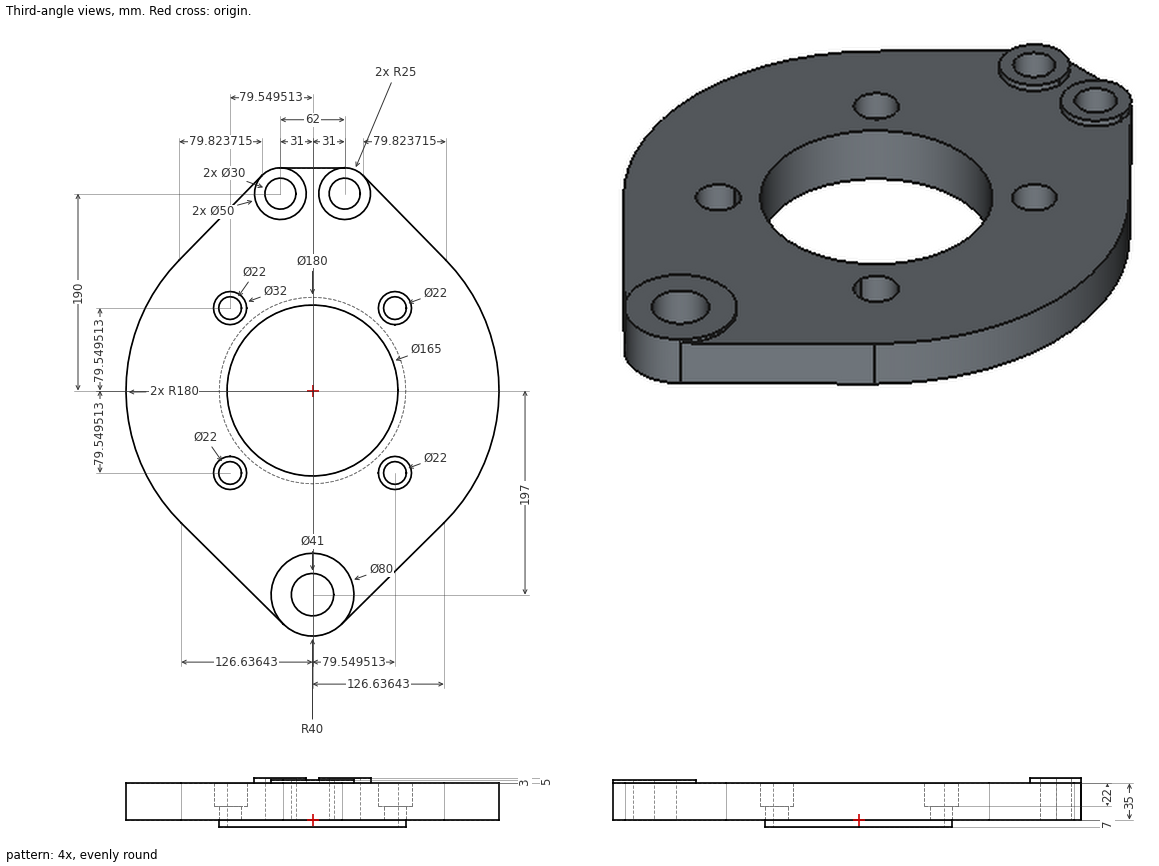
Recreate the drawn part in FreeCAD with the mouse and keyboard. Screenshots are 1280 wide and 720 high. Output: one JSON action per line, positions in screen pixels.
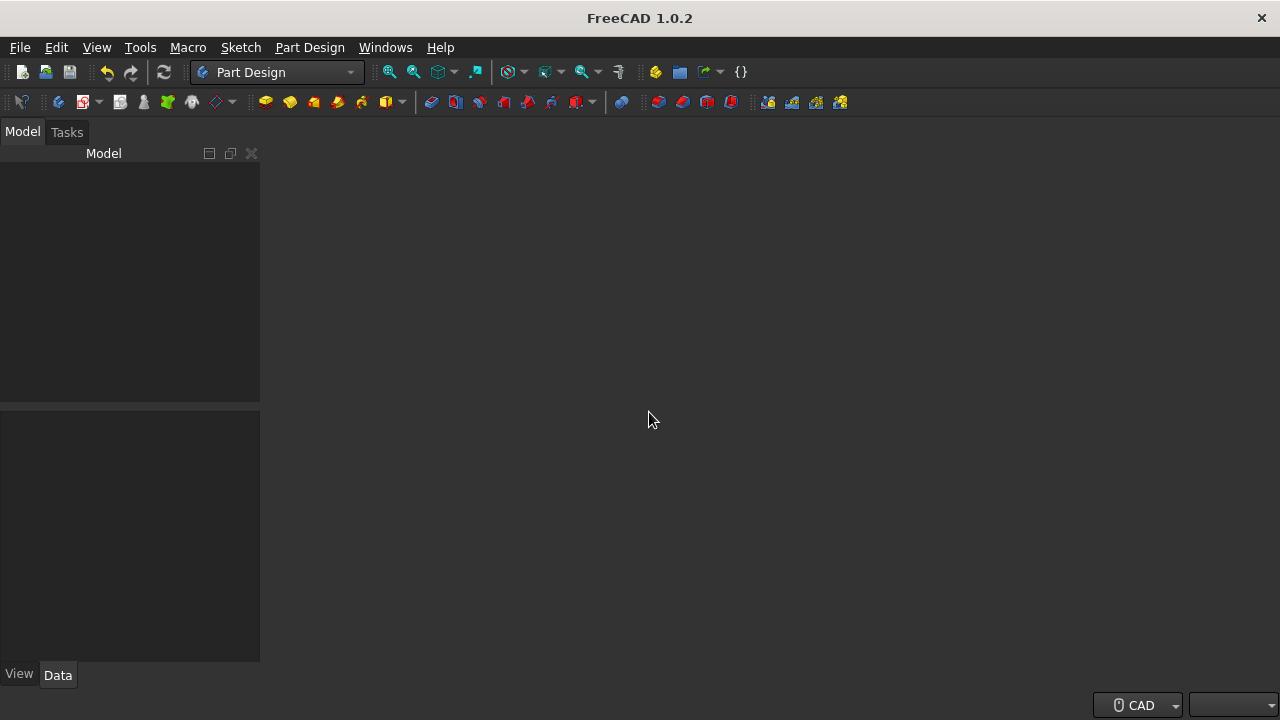
{"action": "key", "text": "ctrl+n"}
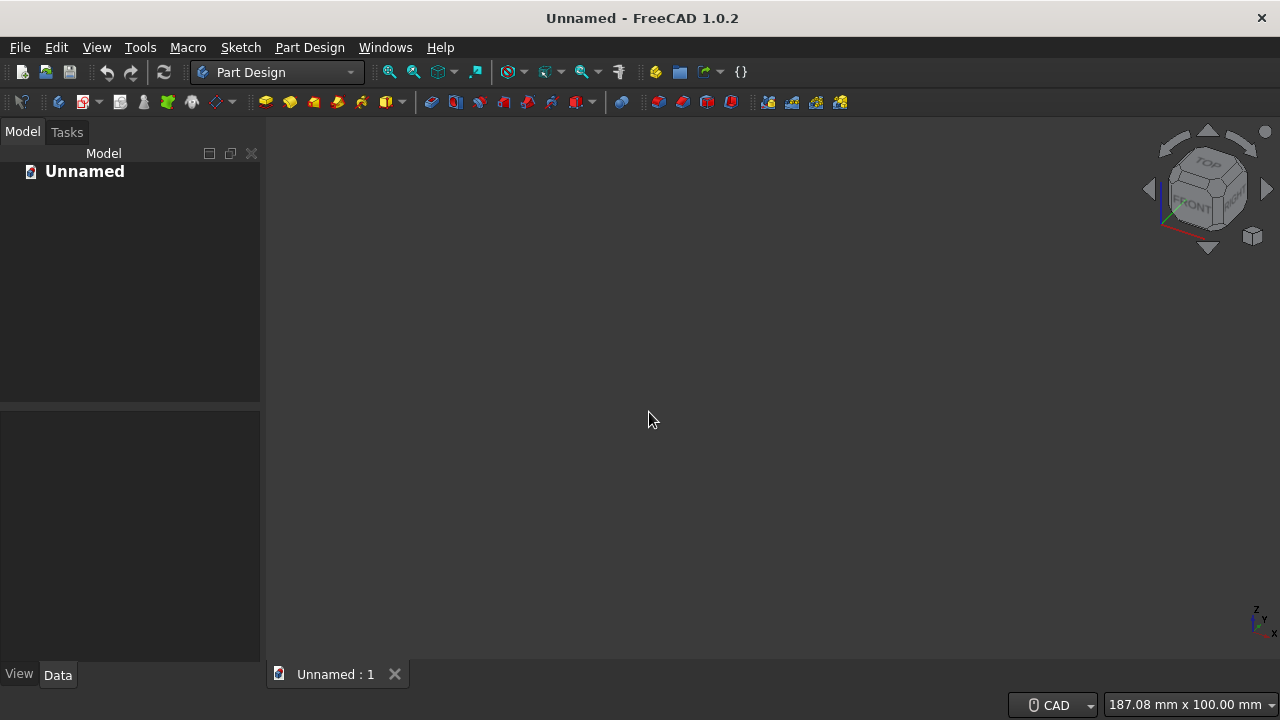
{"action": "left_click", "coordinate": [84, 102]}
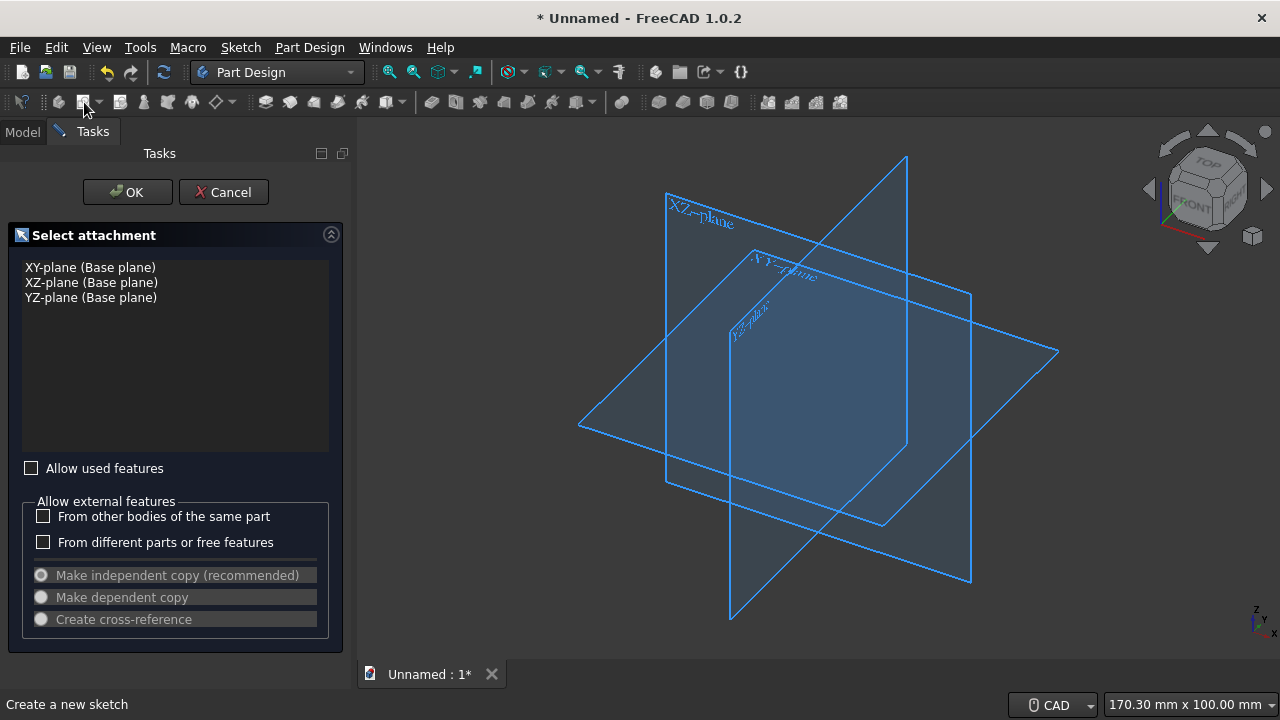
{"action": "left_click", "coordinate": [82, 268]}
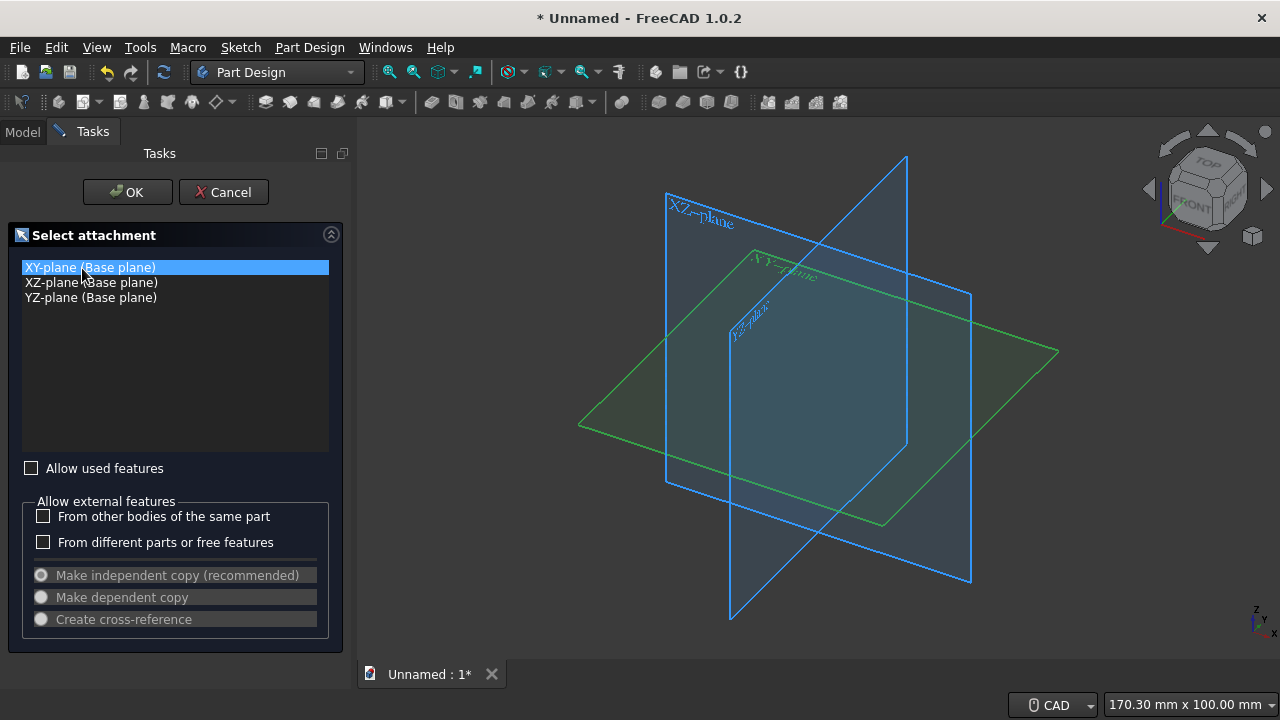
{"action": "left_click", "coordinate": [128, 192]}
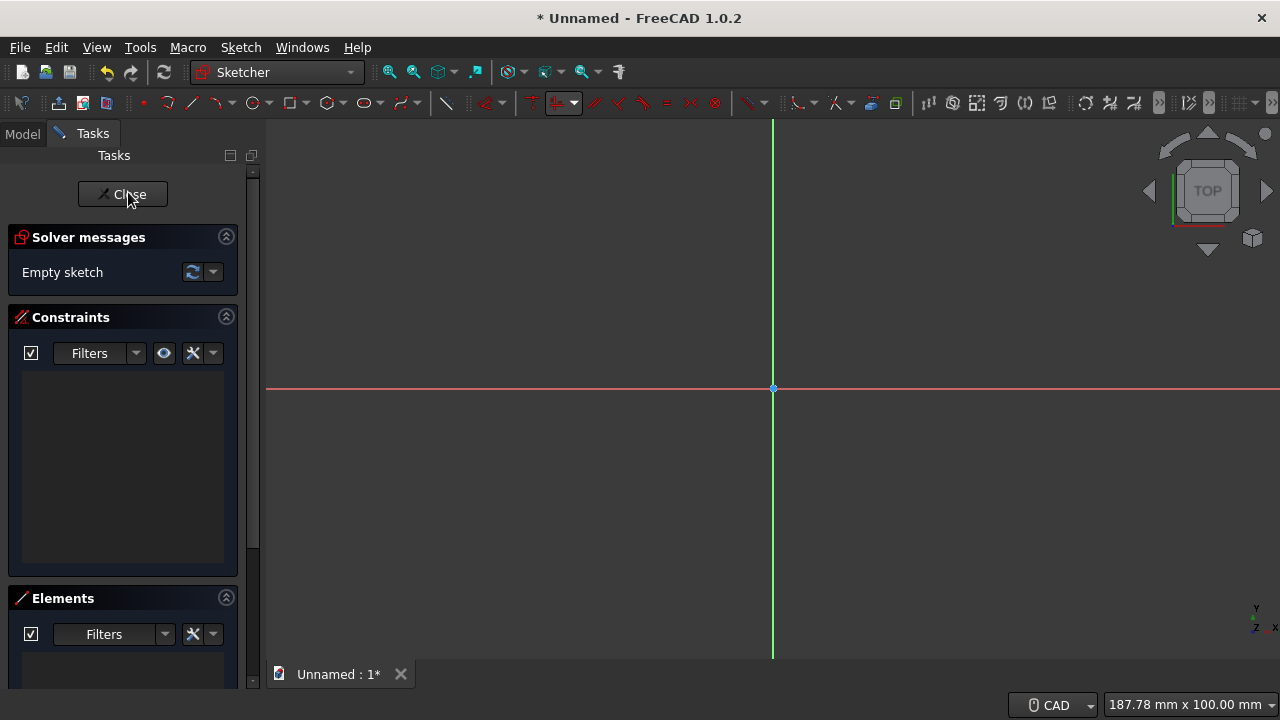
{"action": "scroll", "coordinate": [694, 380], "scroll_direction": "down", "scroll_amount": 10}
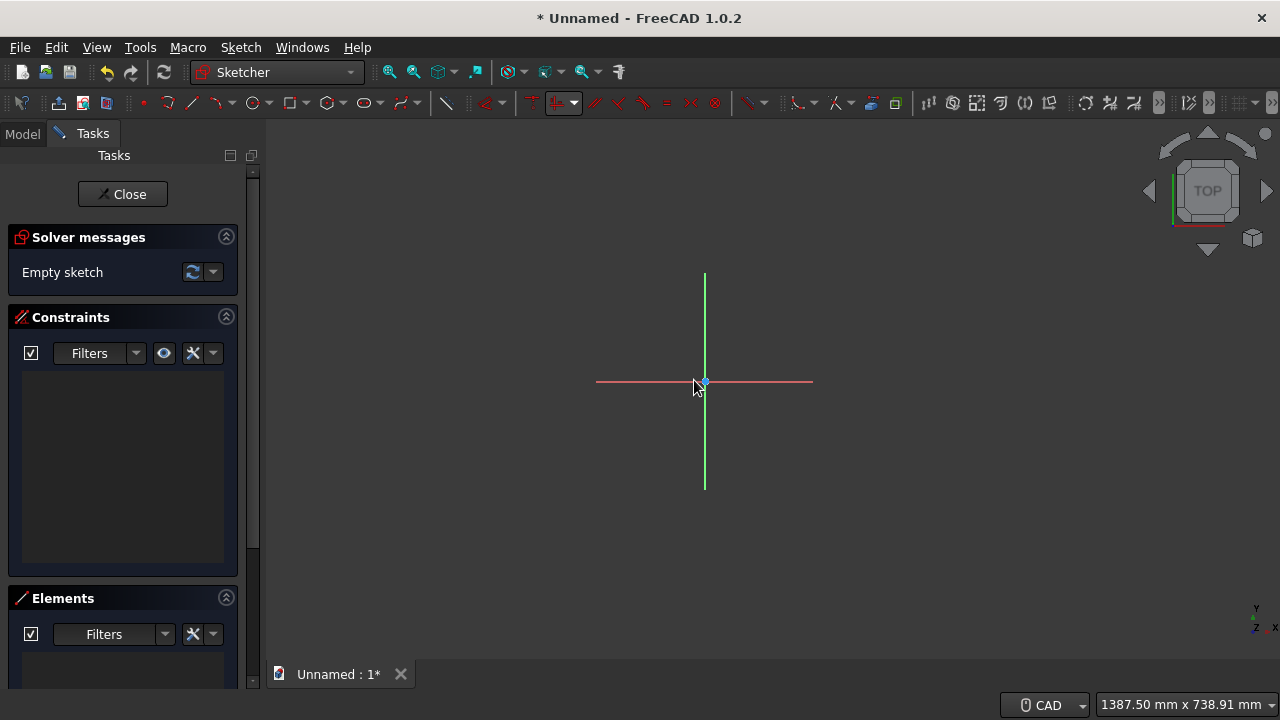
{"action": "key", "text": "g l"}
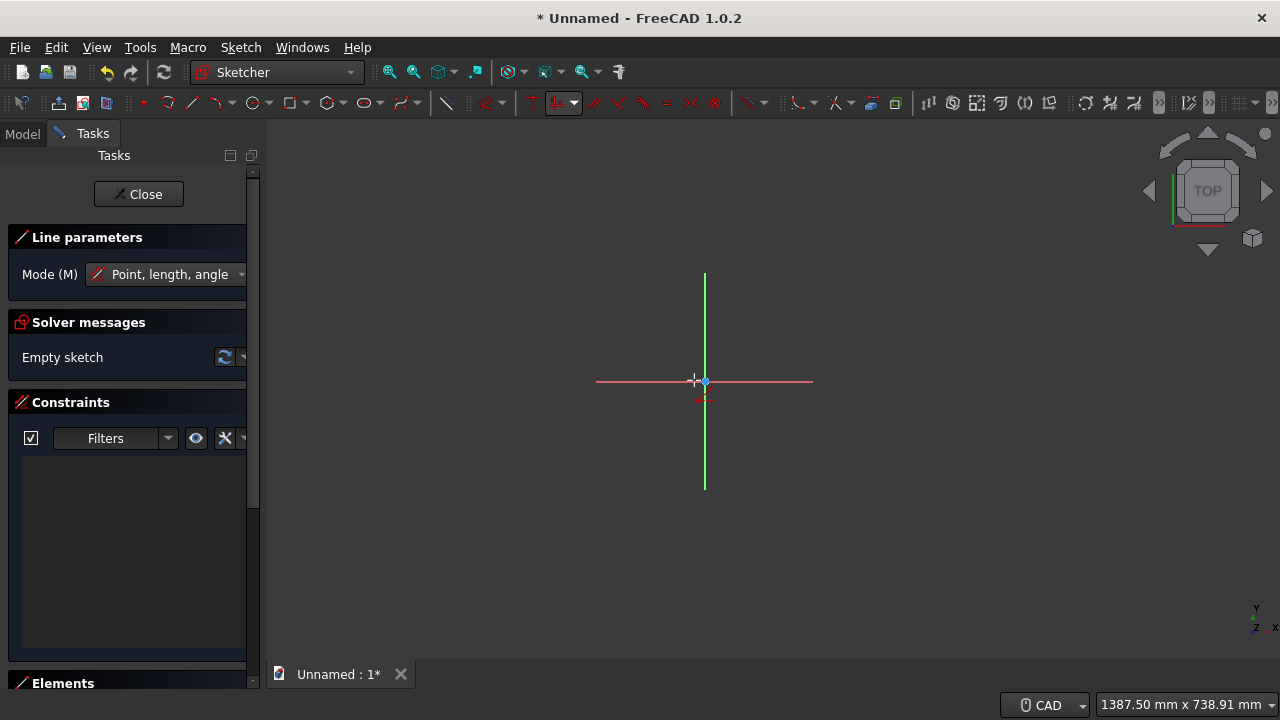
{"action": "left_click", "coordinate": [669, 230]}
{"action": "left_click", "coordinate": [611, 290]}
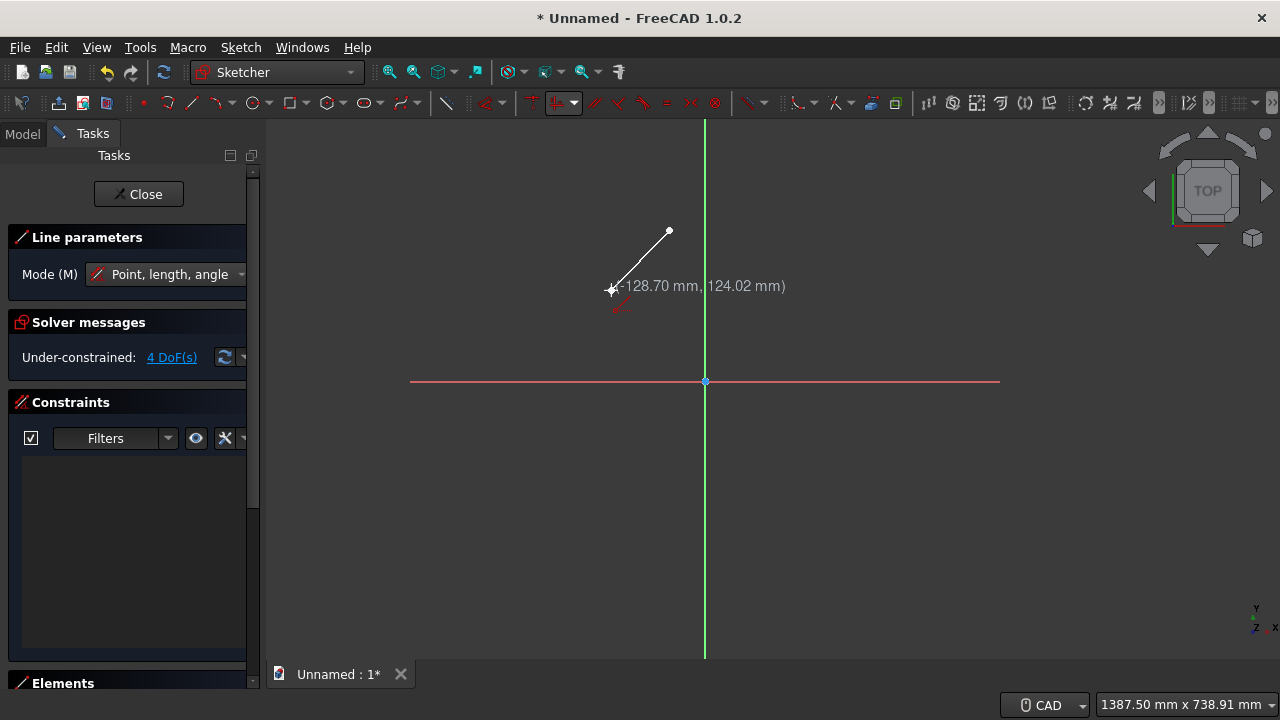
{"action": "left_click", "coordinate": [613, 475]}
{"action": "left_click", "coordinate": [684, 546]}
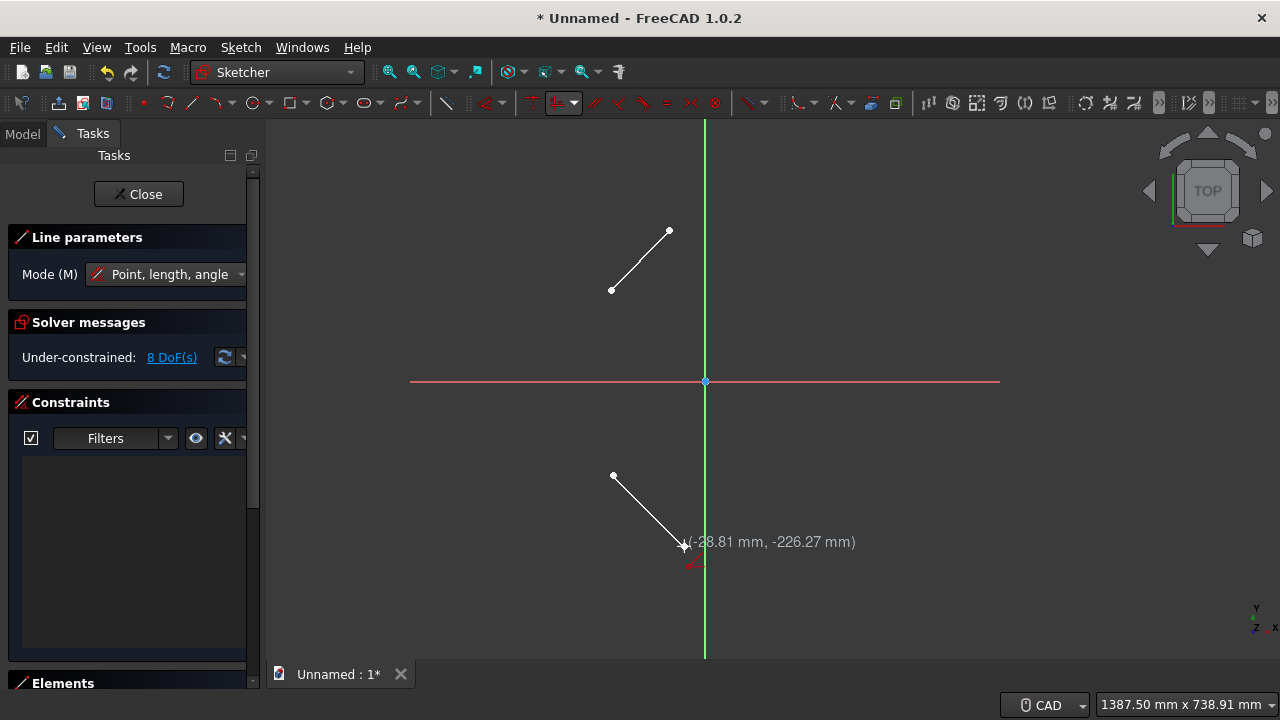
{"action": "left_click", "coordinate": [726, 546]}
{"action": "left_click", "coordinate": [798, 475]}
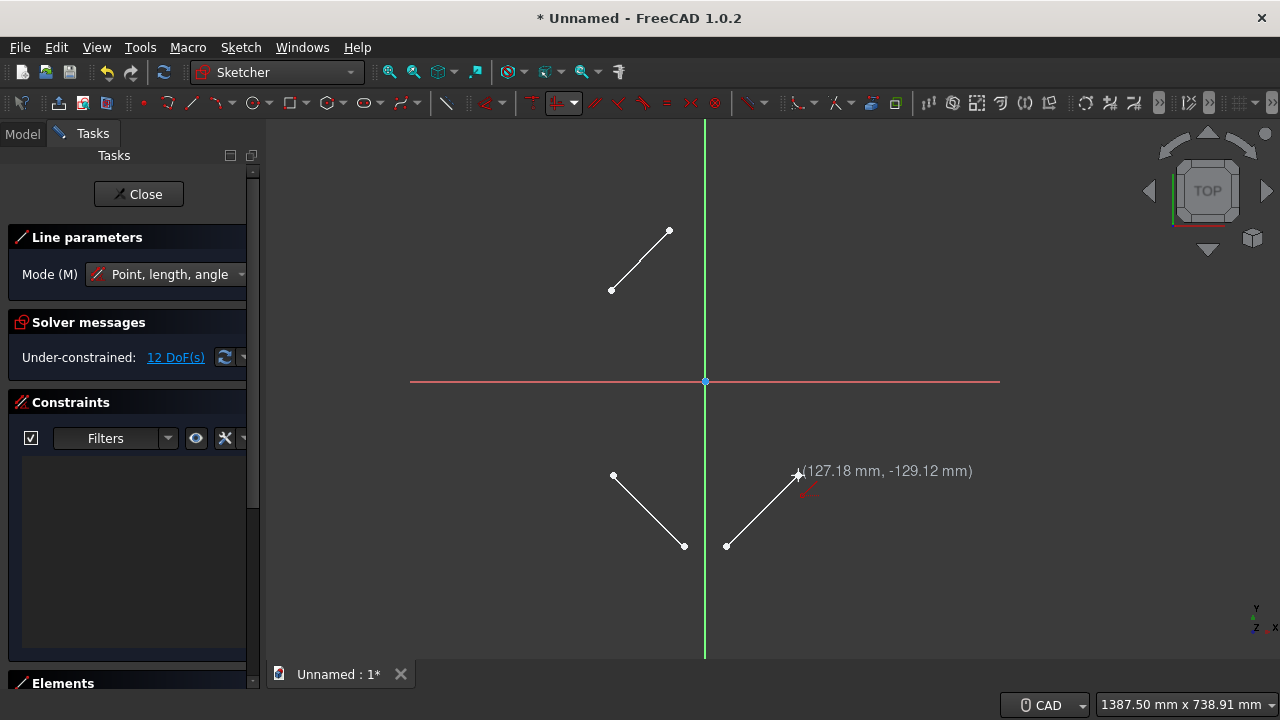
{"action": "left_click", "coordinate": [799, 290]}
{"action": "left_click", "coordinate": [741, 230]}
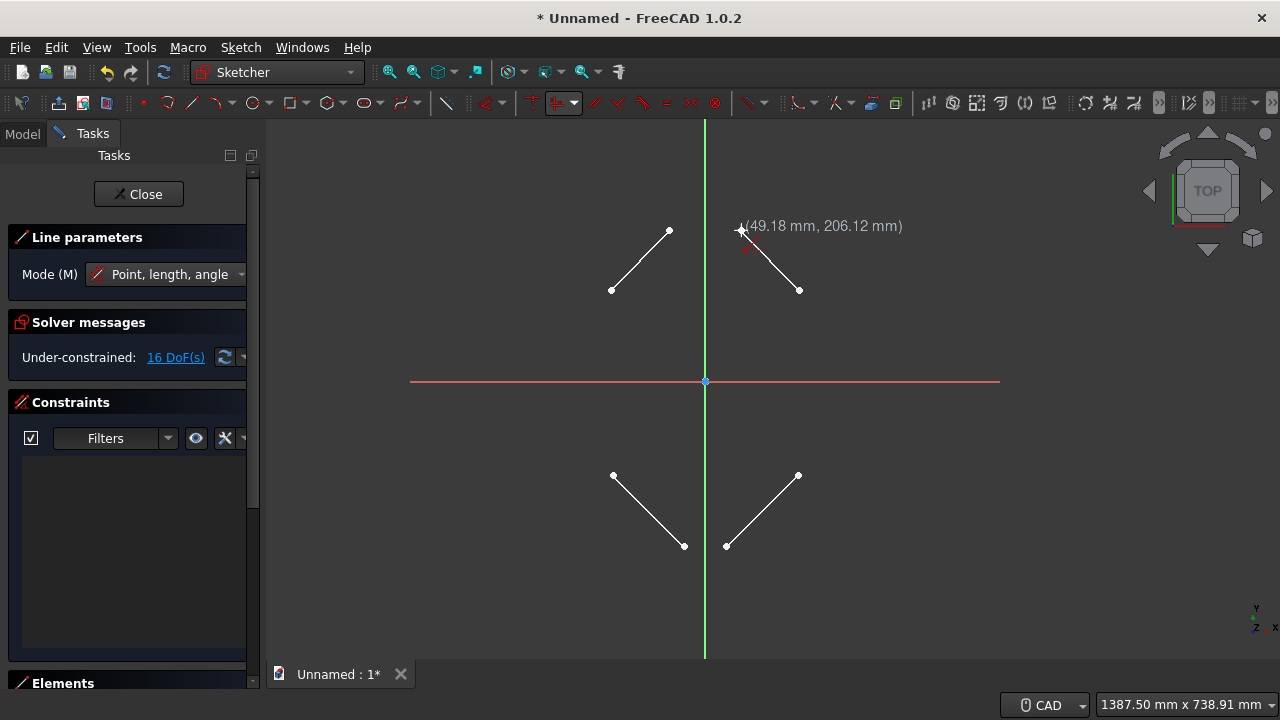
{"action": "left_click", "coordinate": [728, 225]}
{"action": "left_click", "coordinate": [682, 225]}